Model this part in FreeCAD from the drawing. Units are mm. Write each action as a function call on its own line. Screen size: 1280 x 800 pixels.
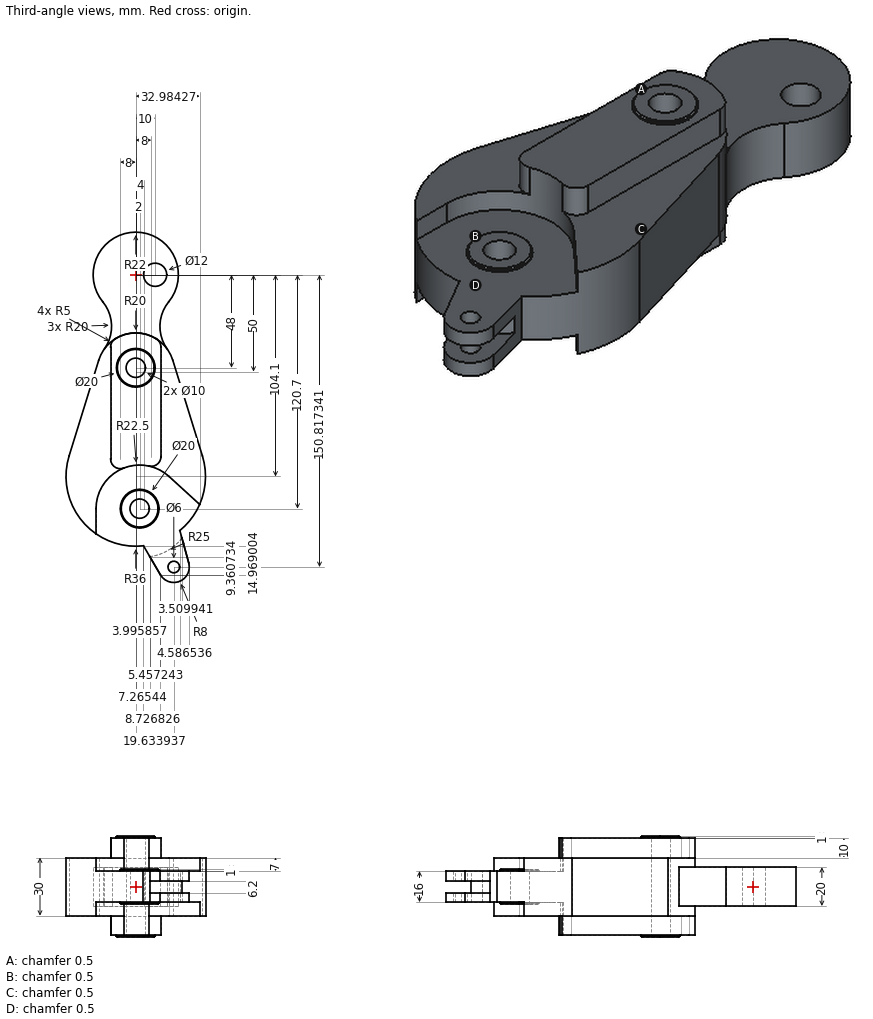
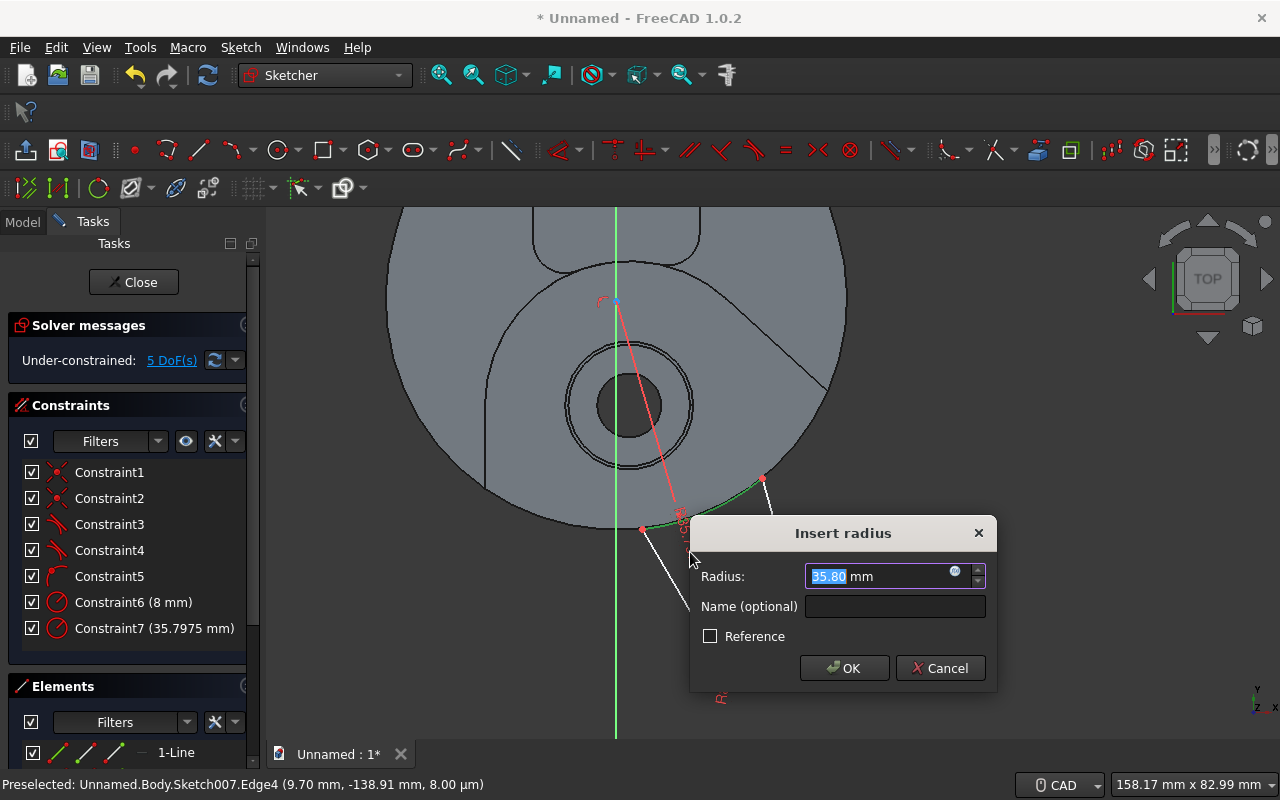
text(36)
key(Return)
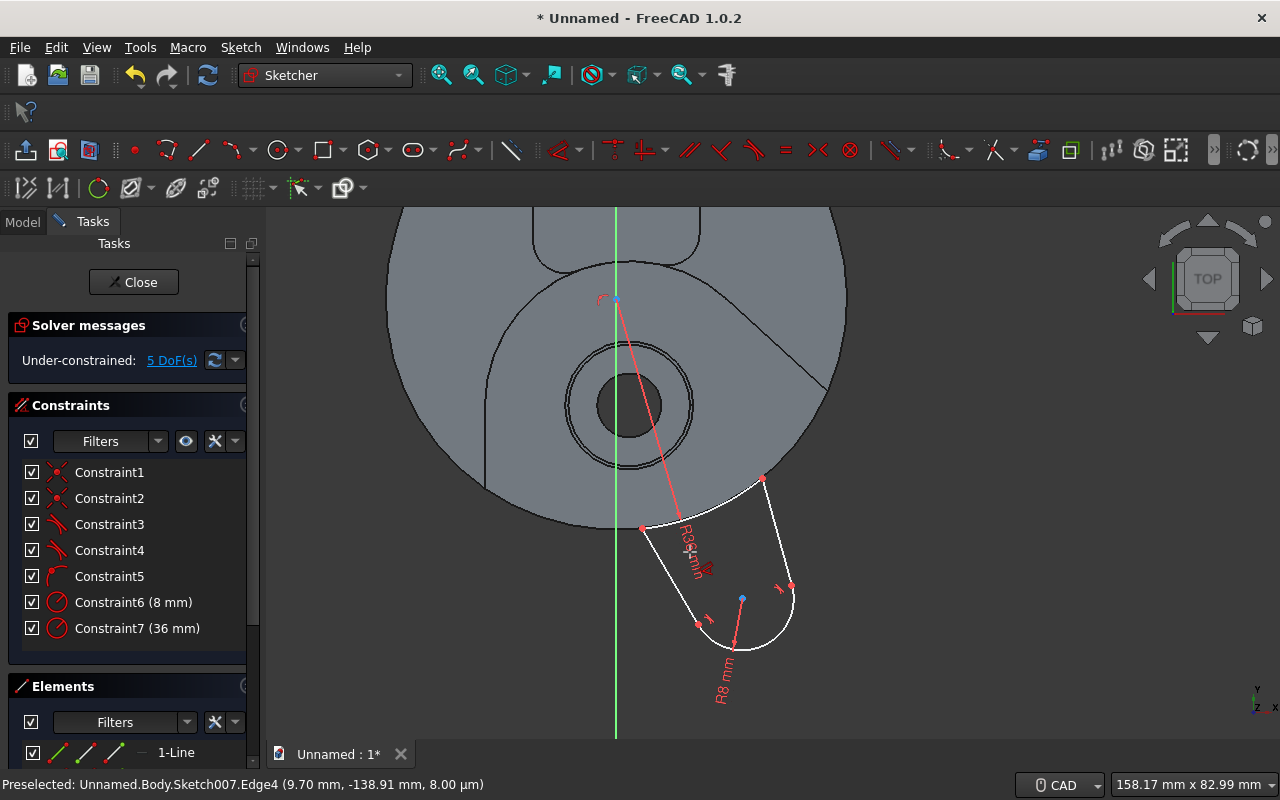
click(616, 300)
click(582, 267)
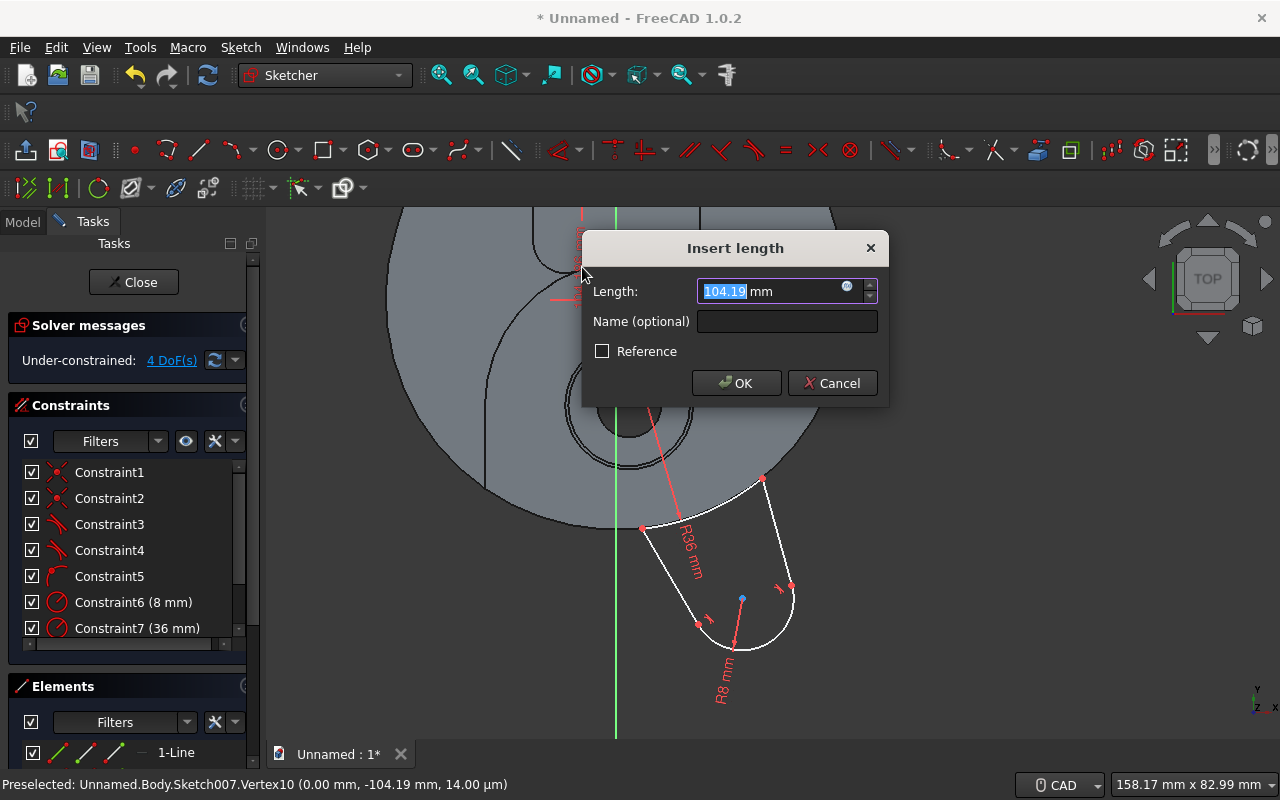
text(104.1)
key(Return)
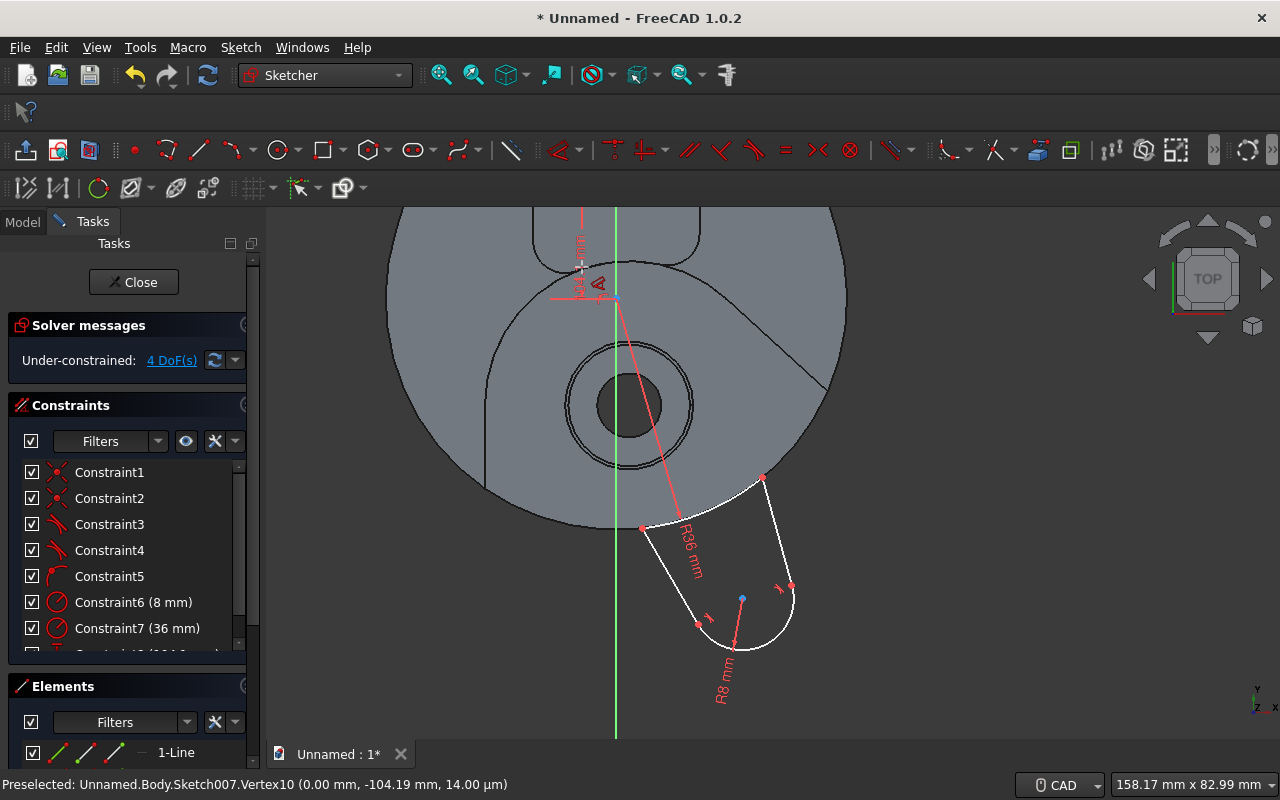
scroll(642, 528, up, 3)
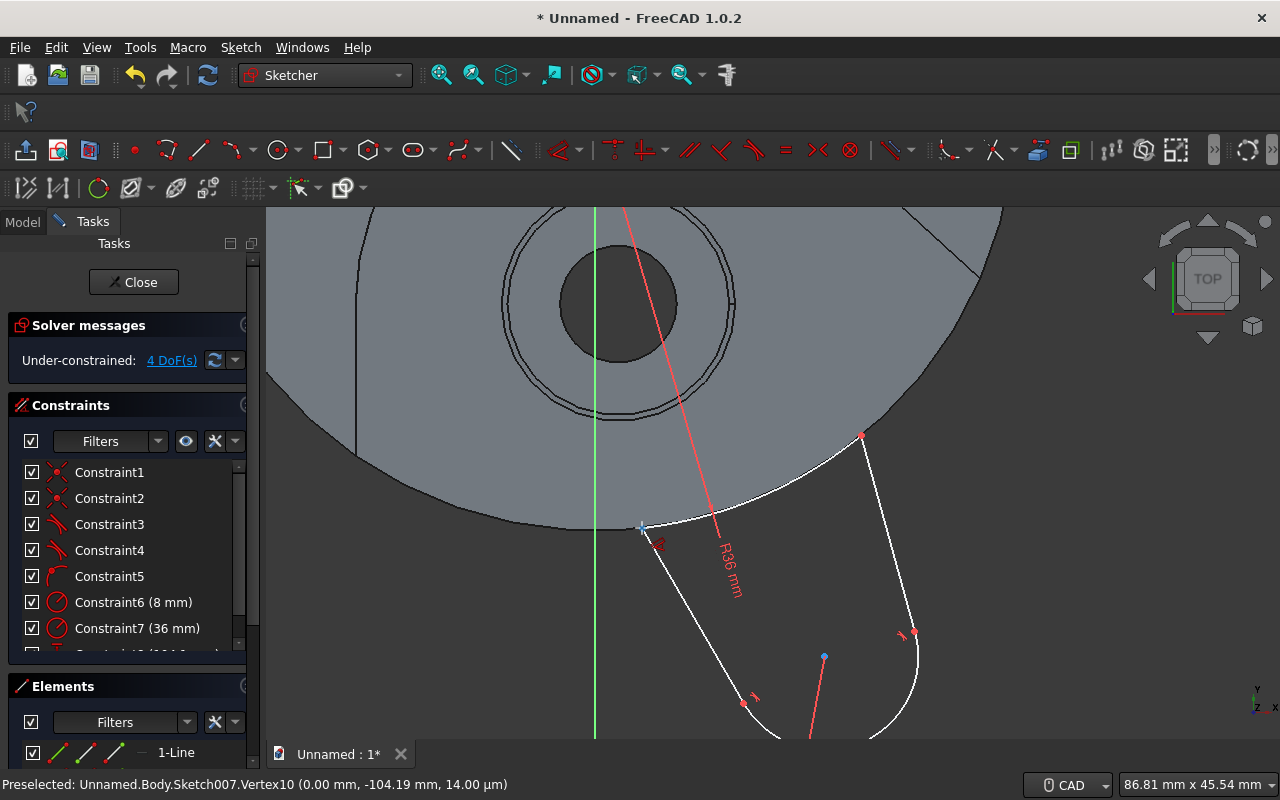
click(642, 528)
click(619, 562)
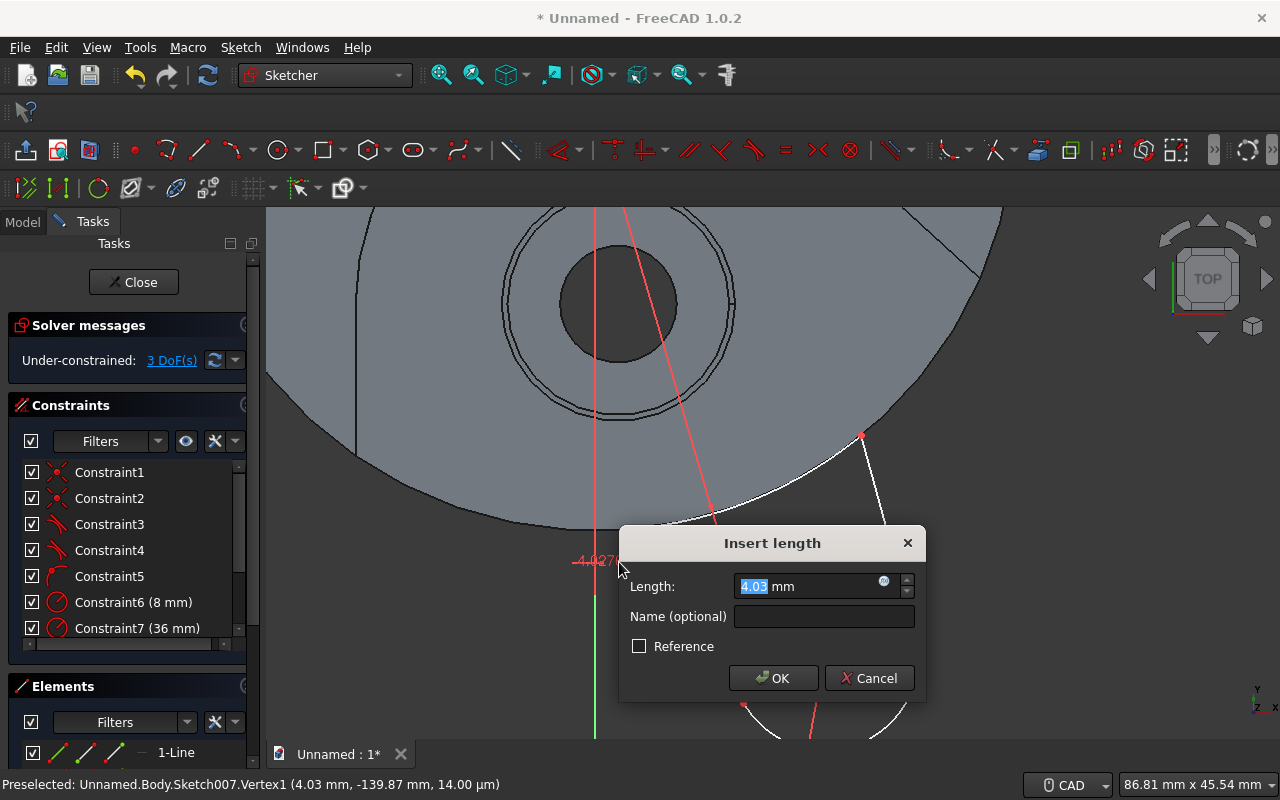
text(3.995857)
key(Return)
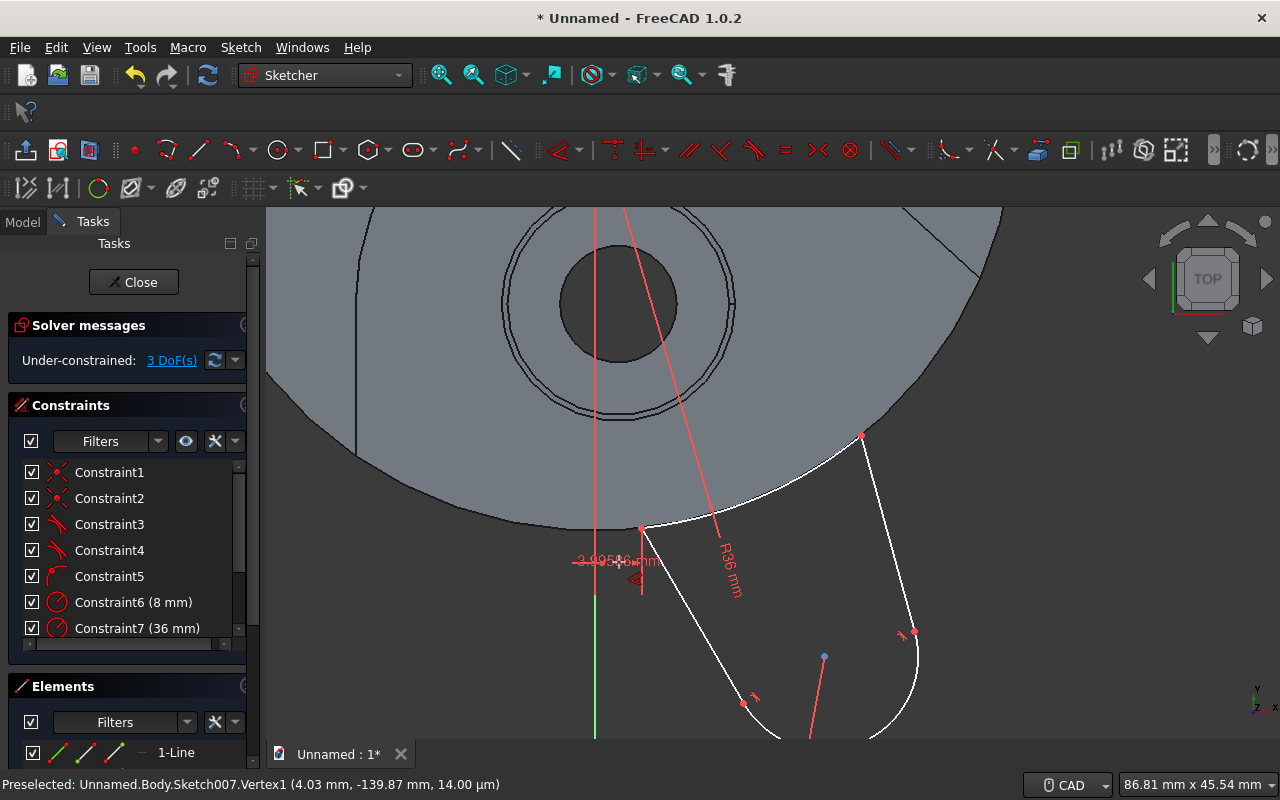
click(672, 581)
click(693, 494)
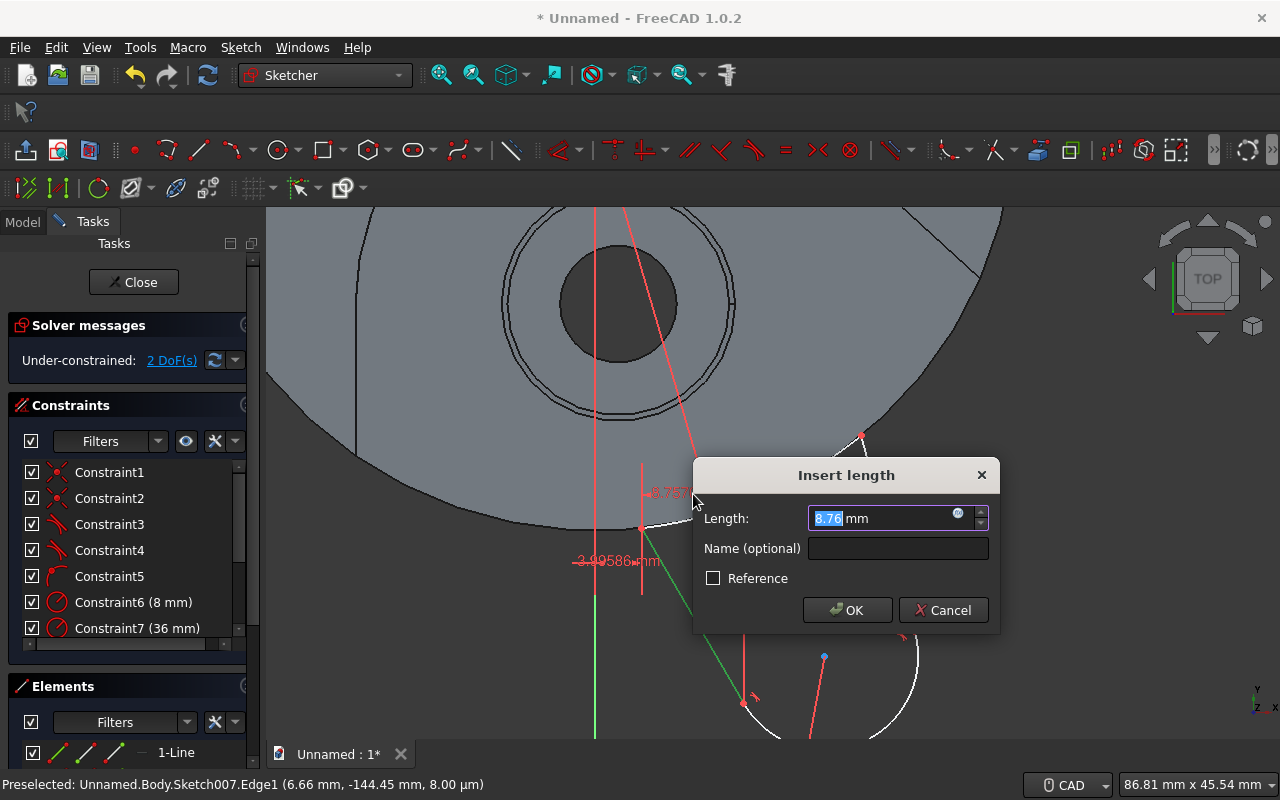
text(8.726826)
key(Return)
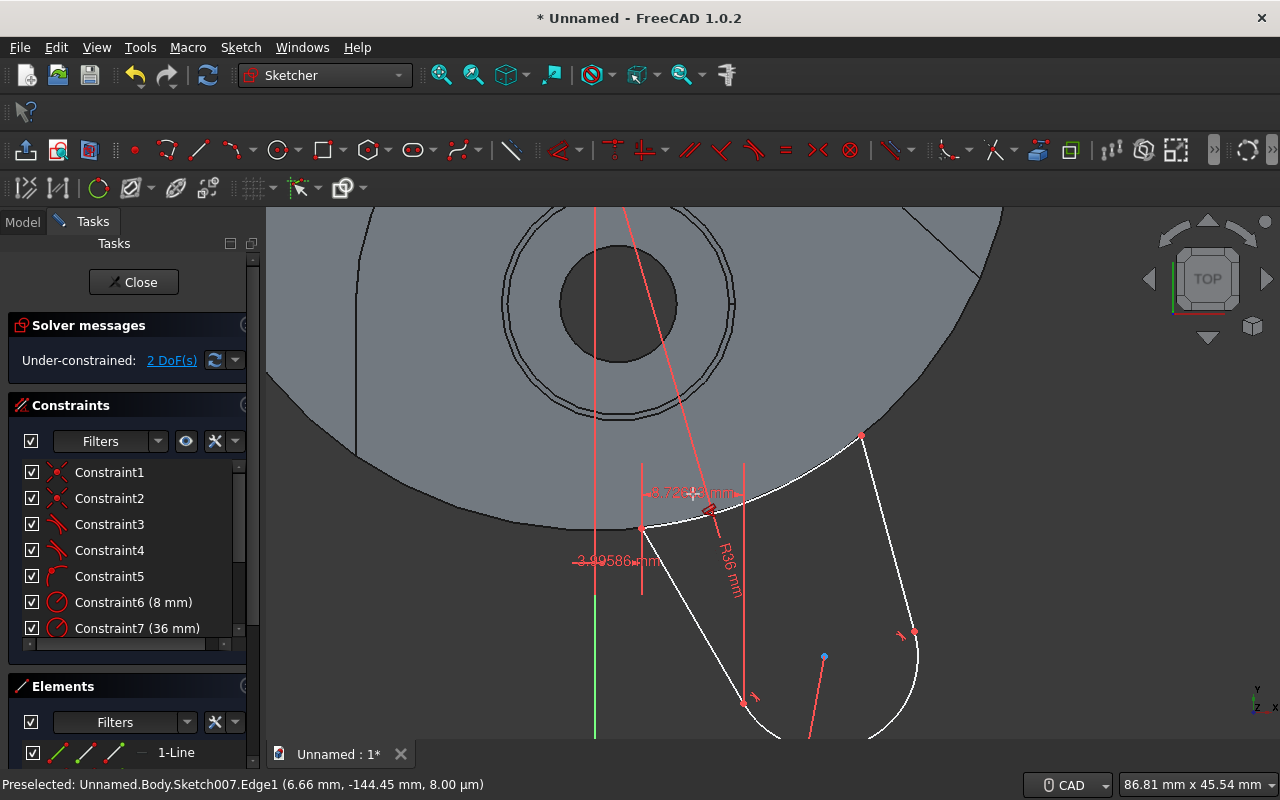
click(899, 573)
click(888, 402)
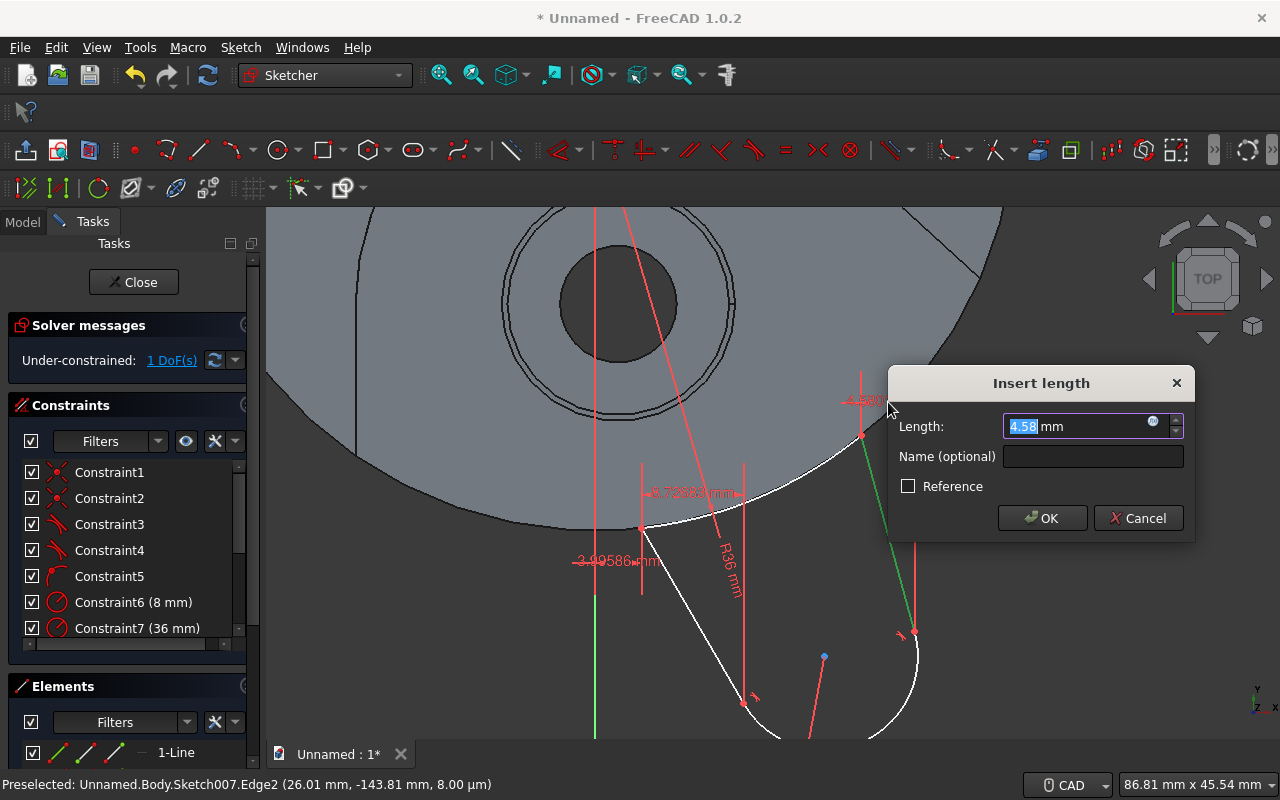
text(4.586536)
key(Return)